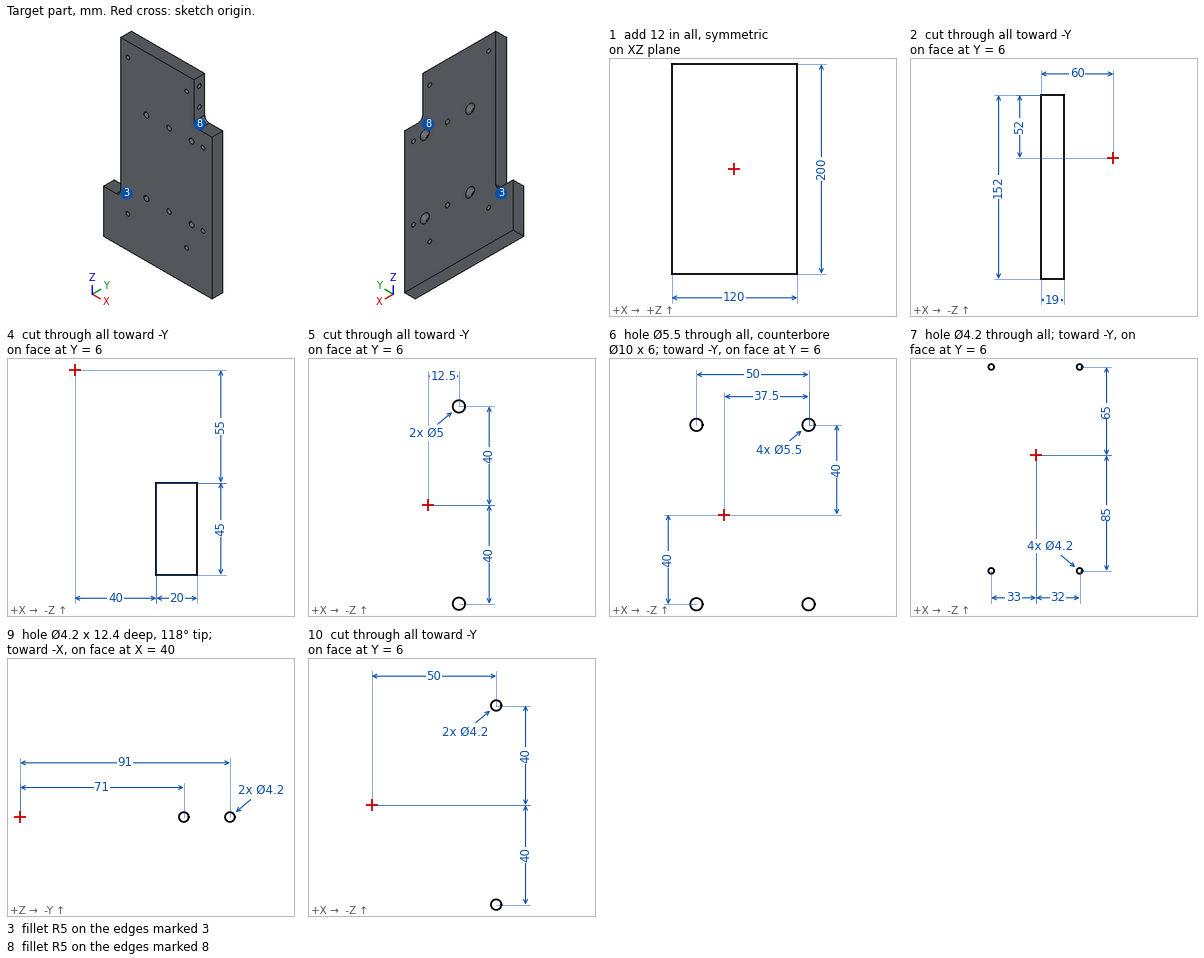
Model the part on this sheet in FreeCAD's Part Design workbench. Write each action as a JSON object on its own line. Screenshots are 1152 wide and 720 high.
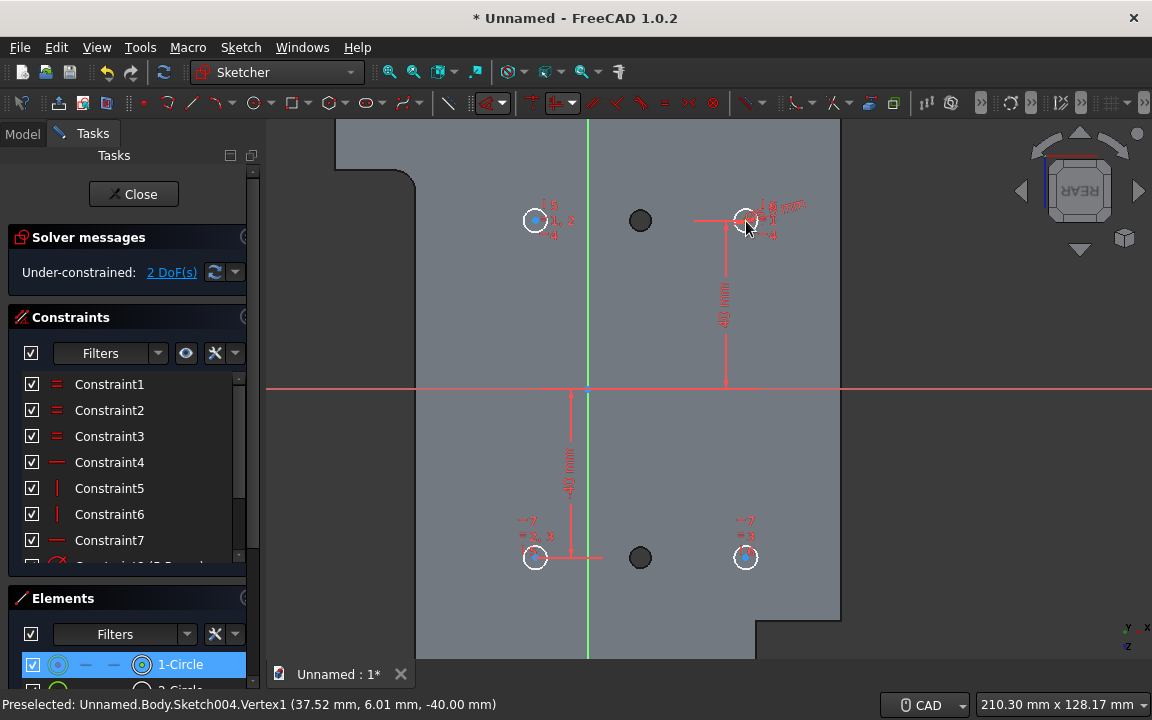
{"action": "left_click", "coordinate": [535, 221]}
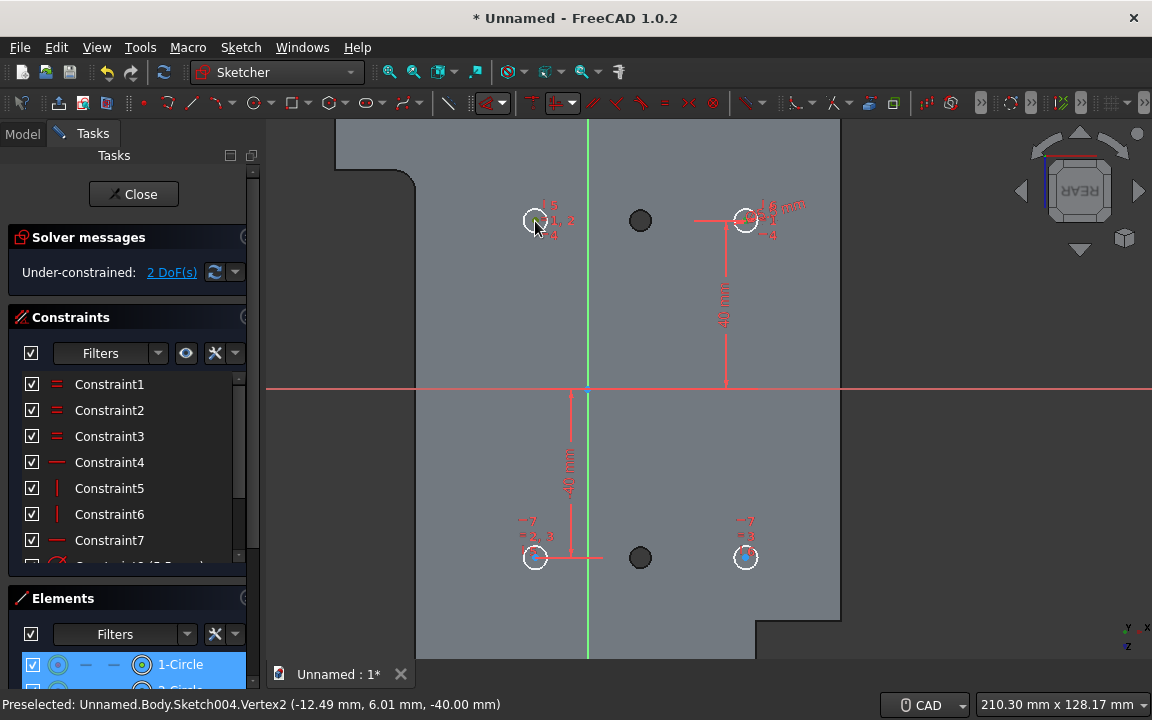
{"action": "left_click", "coordinate": [504, 104]}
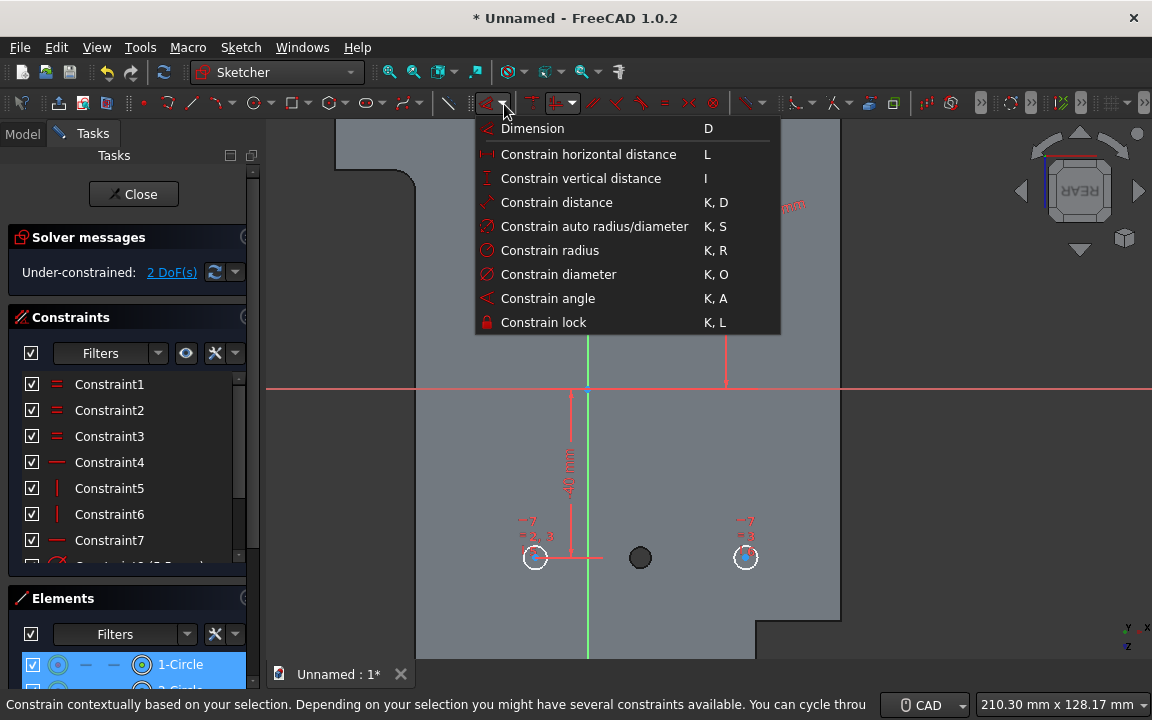
{"action": "left_click", "coordinate": [628, 154]}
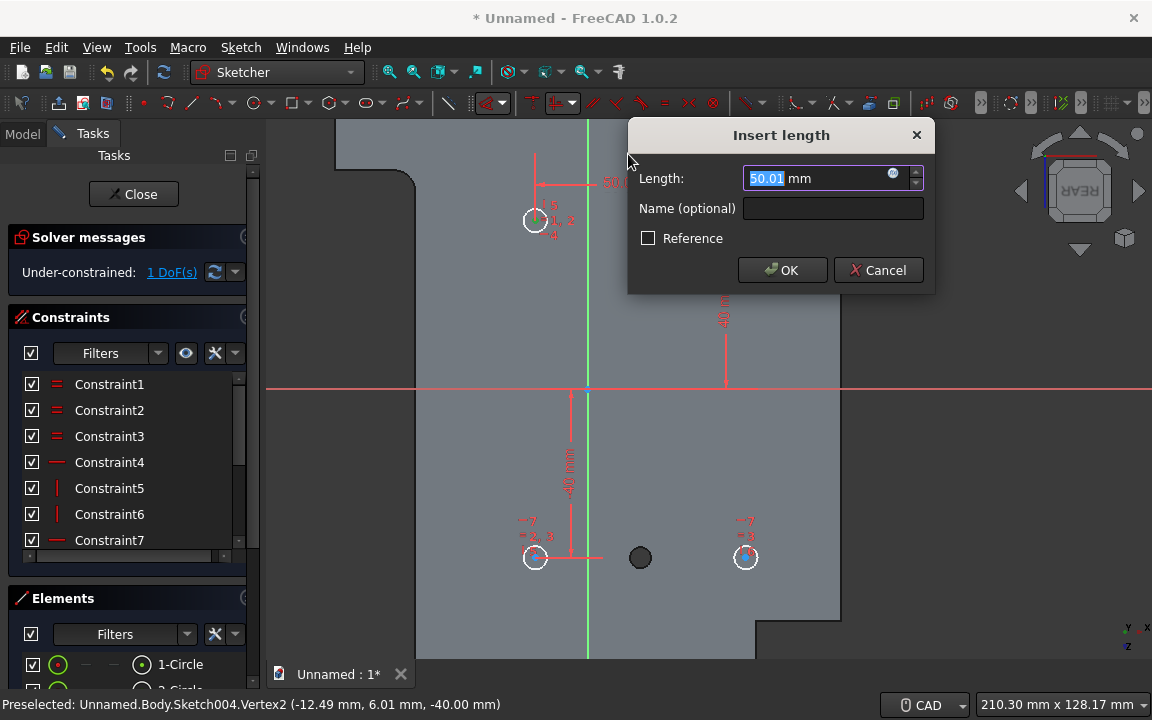
{"action": "type", "text": "50"}
{"action": "key", "text": "Return"}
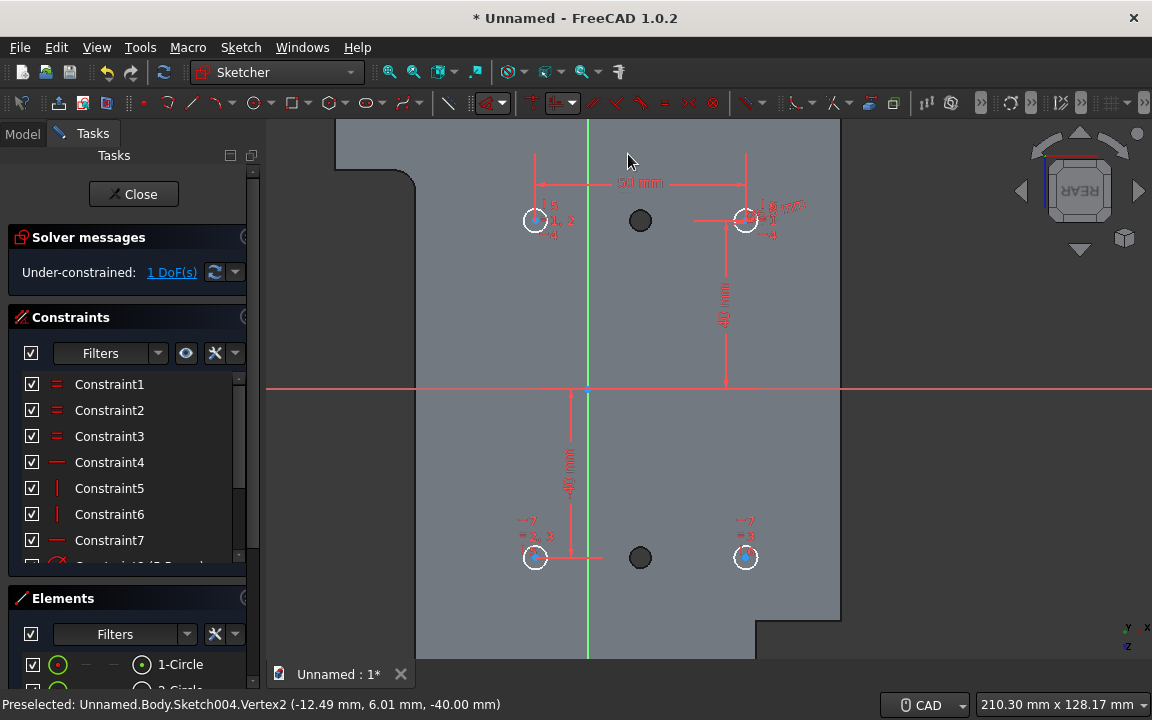
{"action": "left_click", "coordinate": [746, 221]}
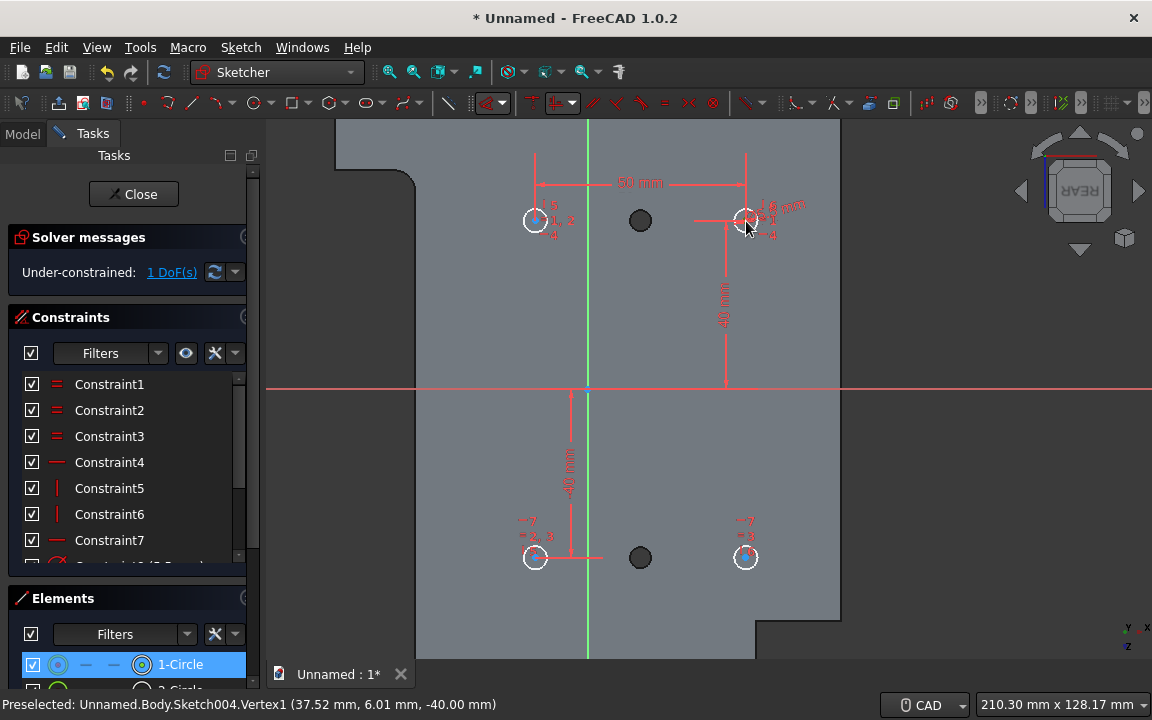
{"action": "key", "text": "l"}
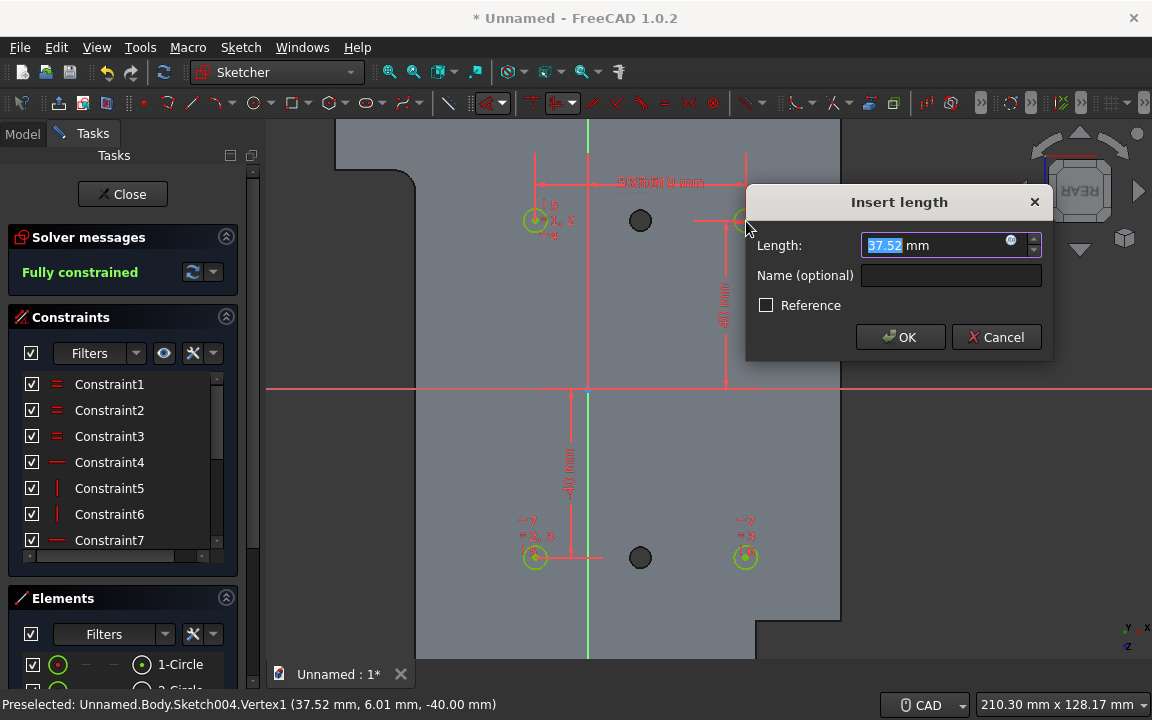
{"action": "type", "text": "37.5"}
{"action": "key", "text": "Return"}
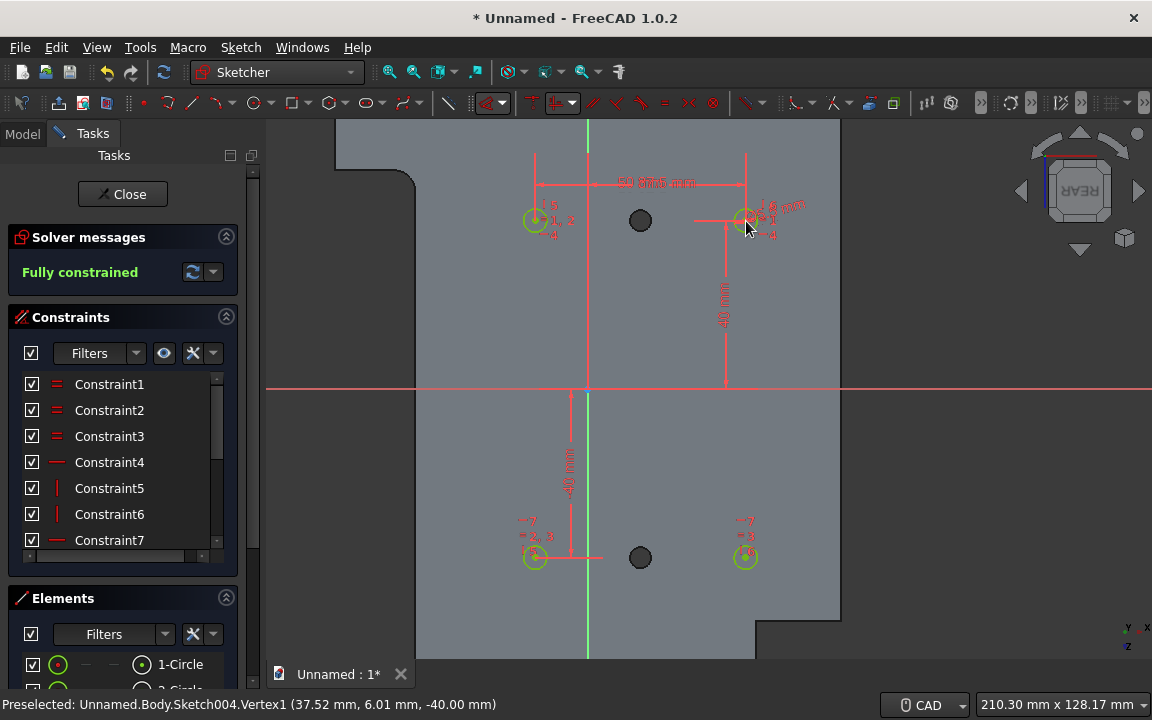
{"action": "left_click", "coordinate": [123, 194]}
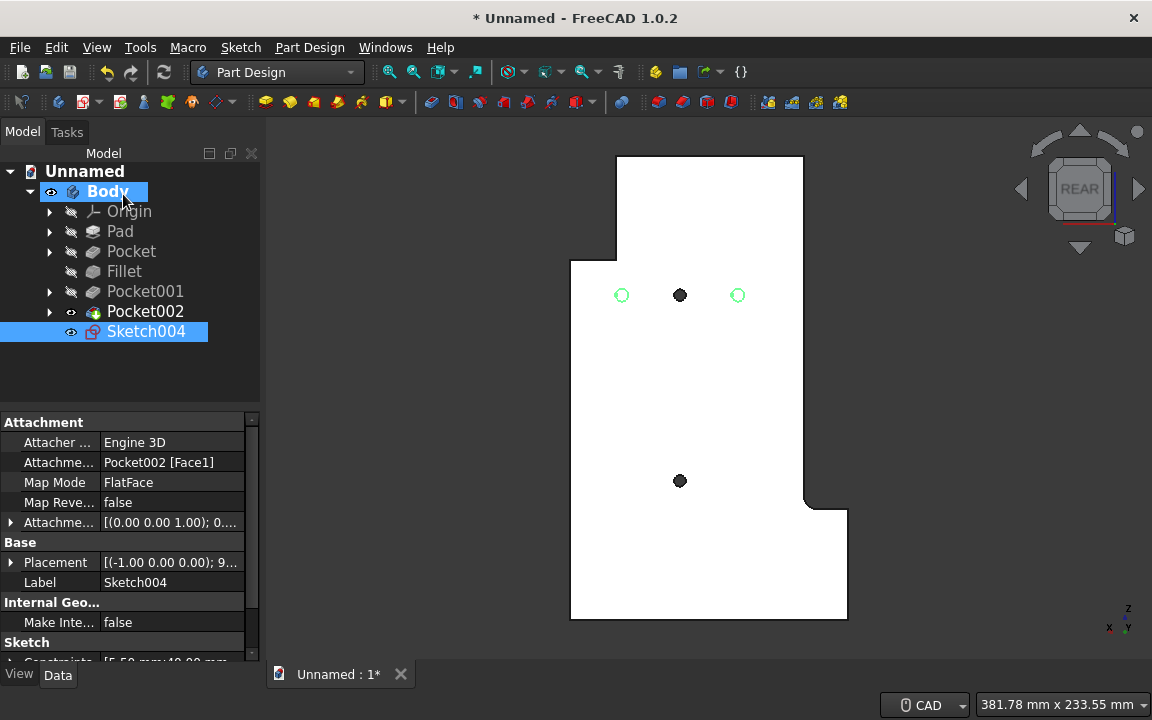
{"action": "left_click", "coordinate": [456, 102]}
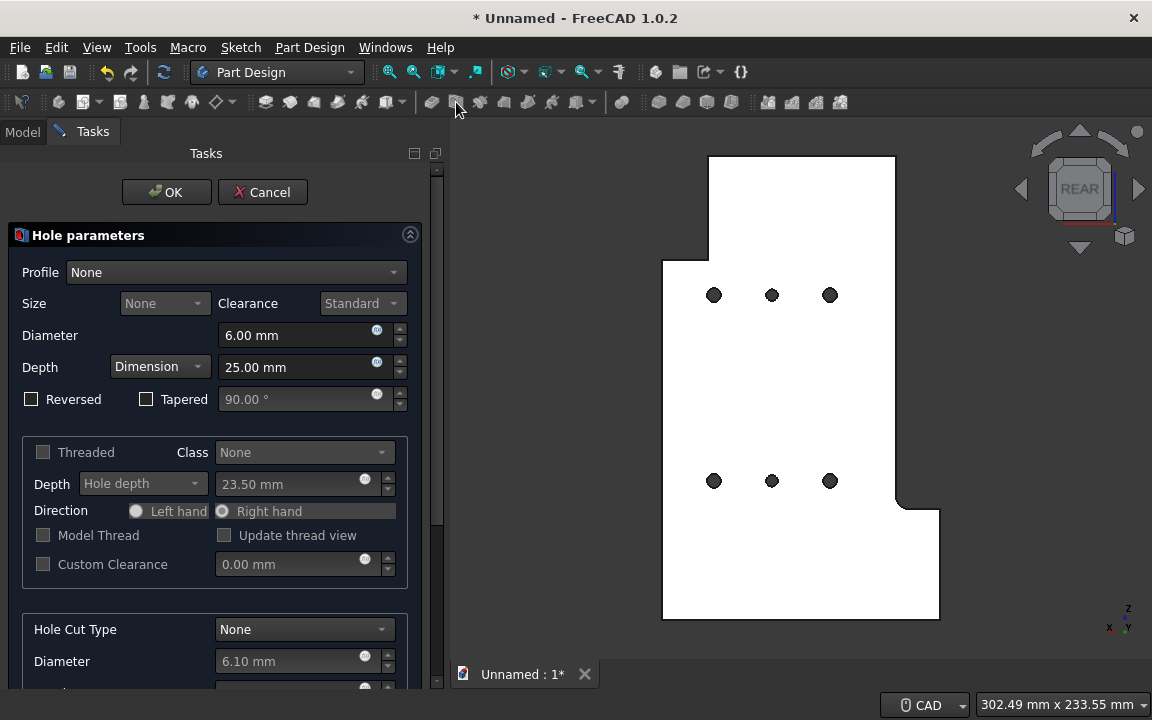
{"action": "triple_click", "coordinate": [305, 335]}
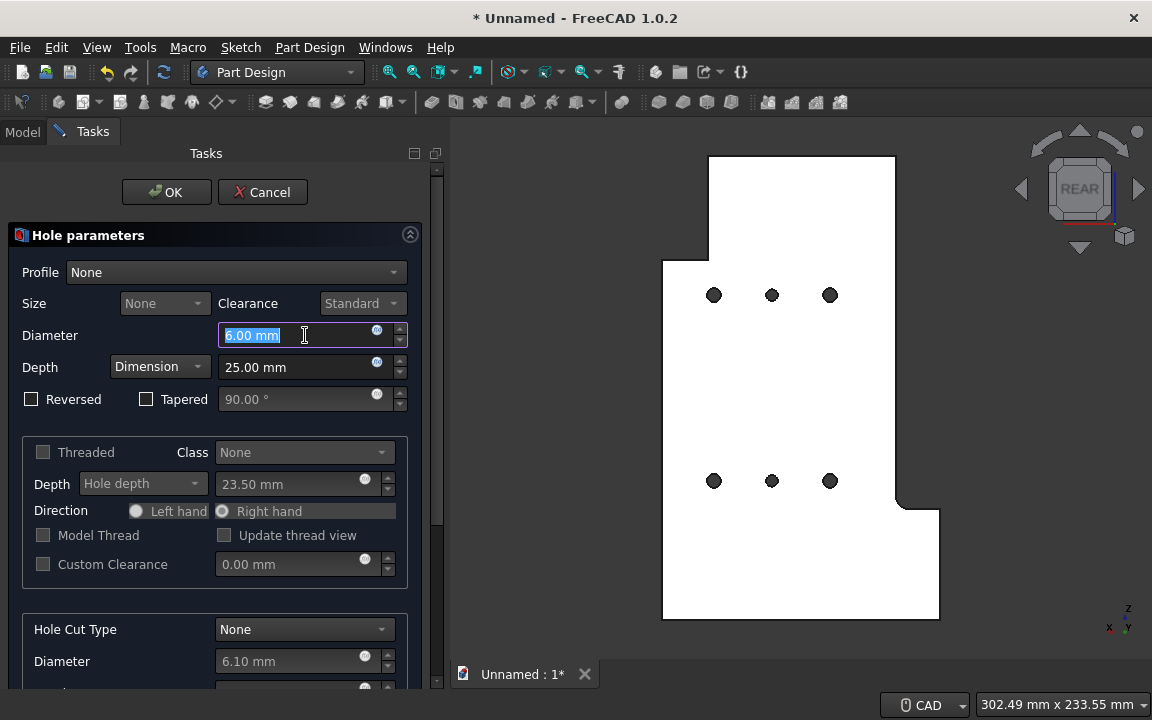
{"action": "type", "text": "5.5"}
{"action": "key", "text": "Tab"}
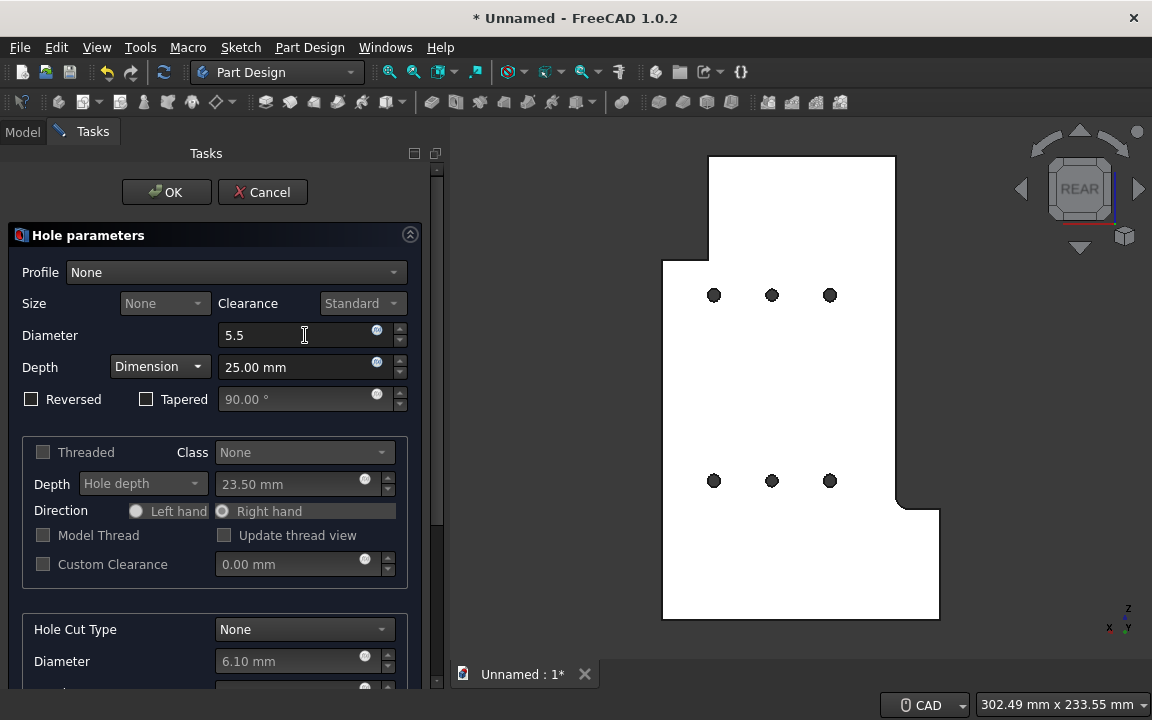
{"action": "left_click", "coordinate": [161, 366]}